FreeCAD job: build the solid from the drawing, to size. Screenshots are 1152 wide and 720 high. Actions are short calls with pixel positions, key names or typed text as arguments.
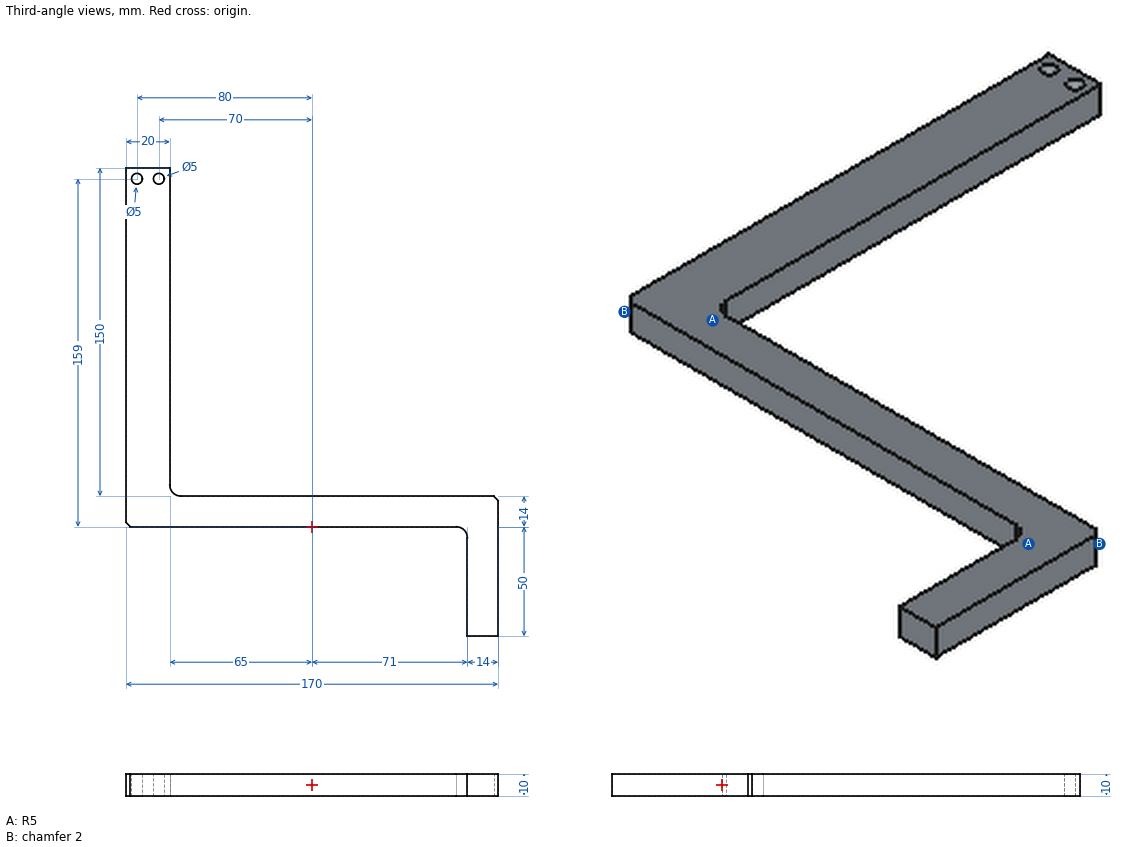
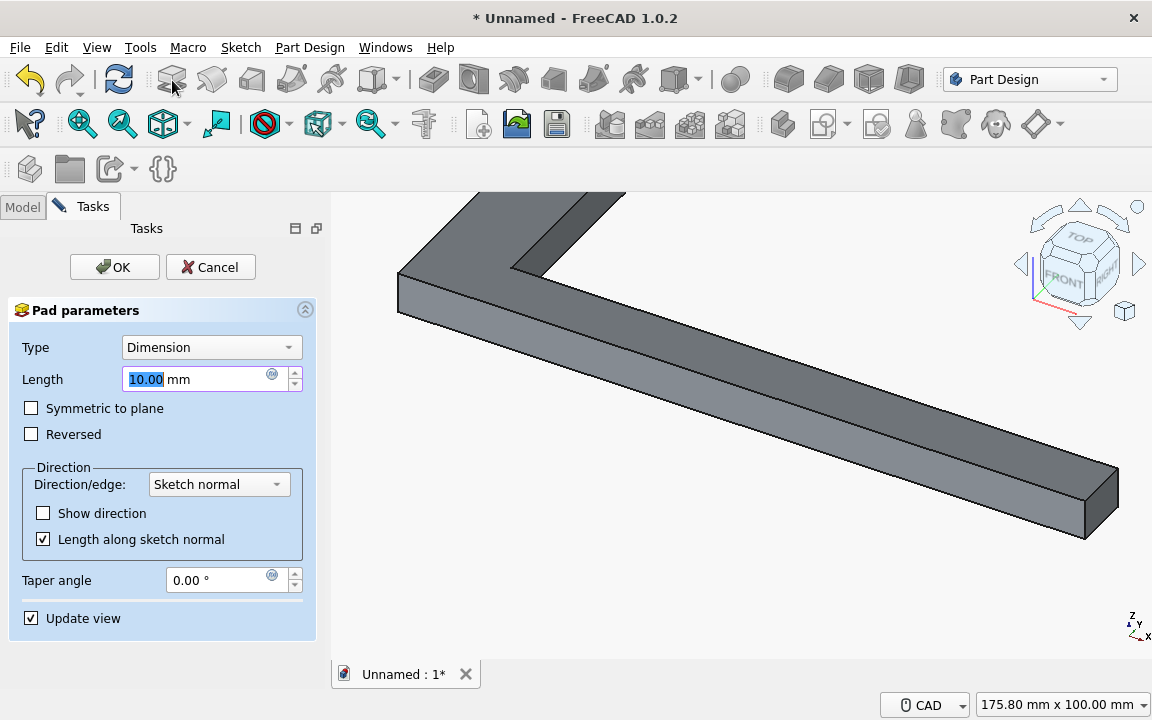
text(10)
key(Tab)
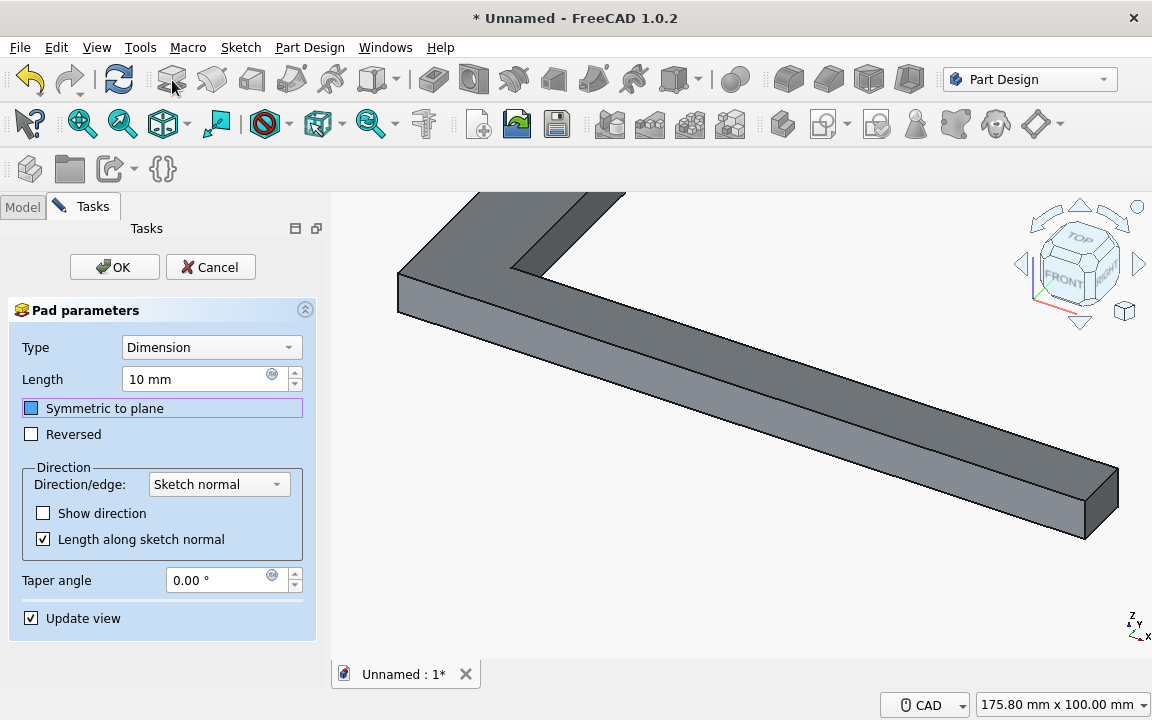
click(30, 408)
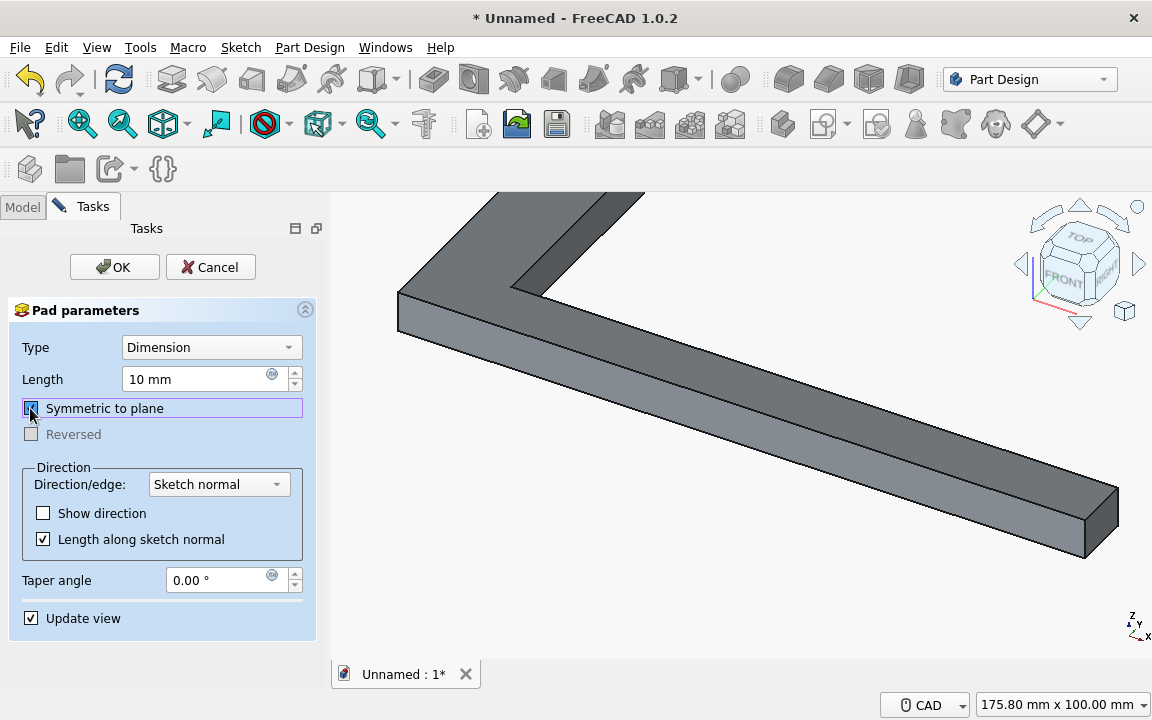
click(115, 267)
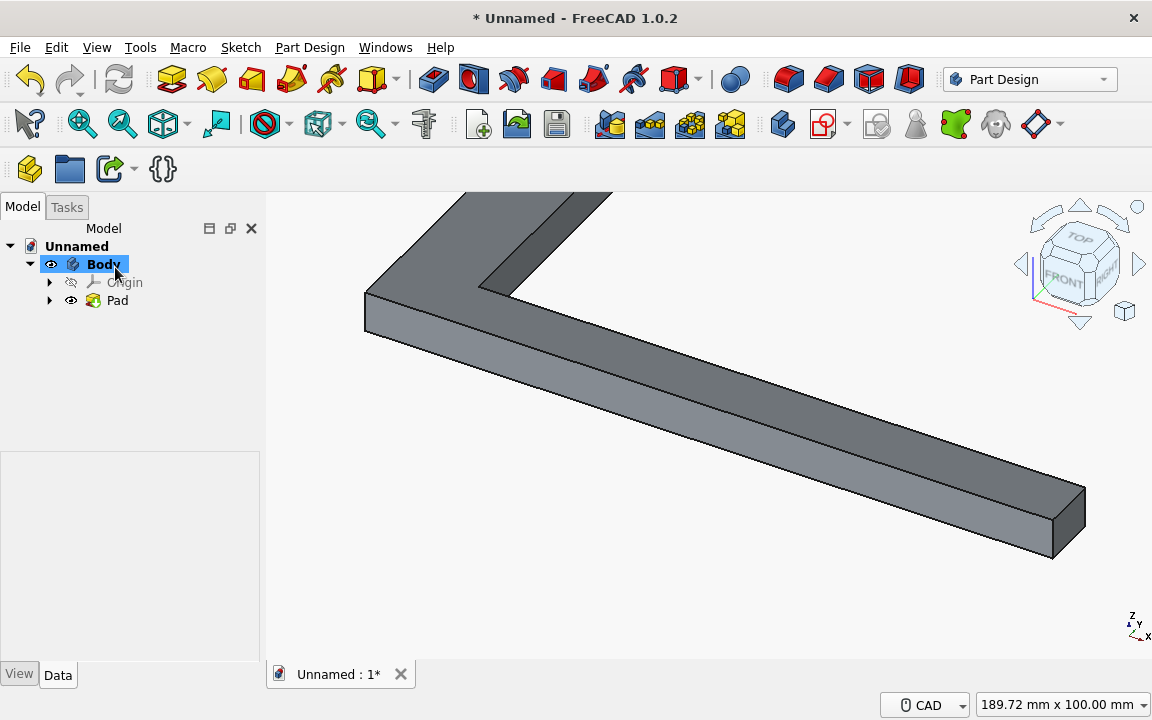
click(84, 124)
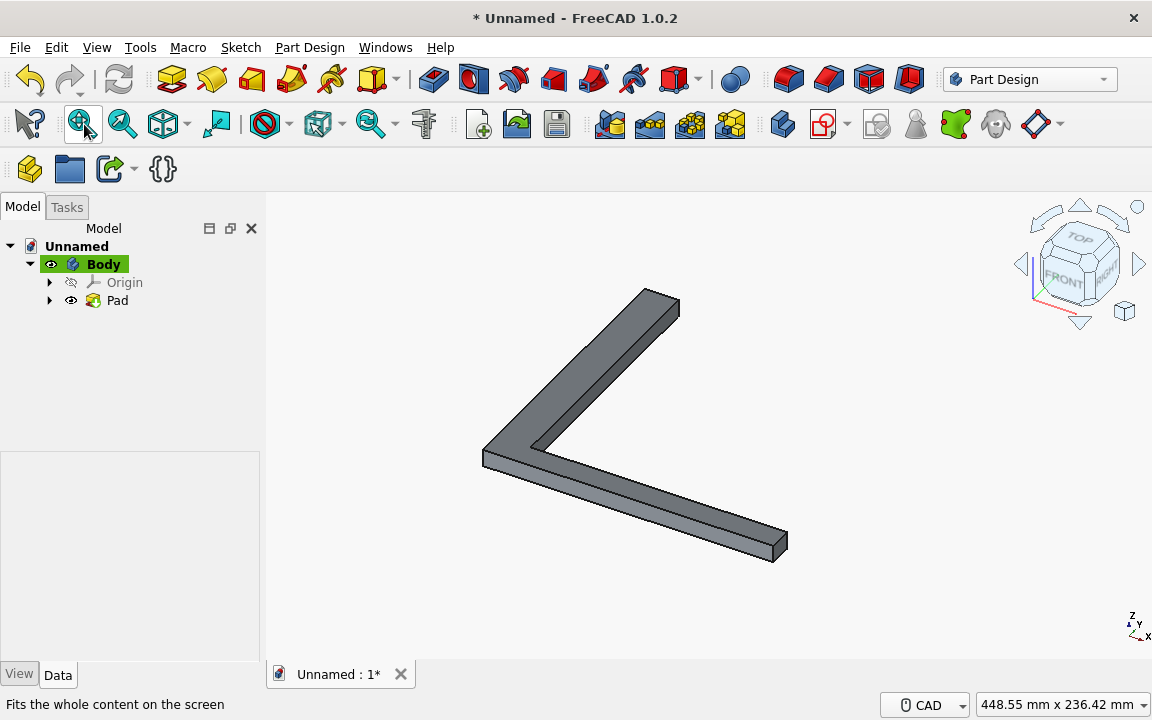
click(515, 444)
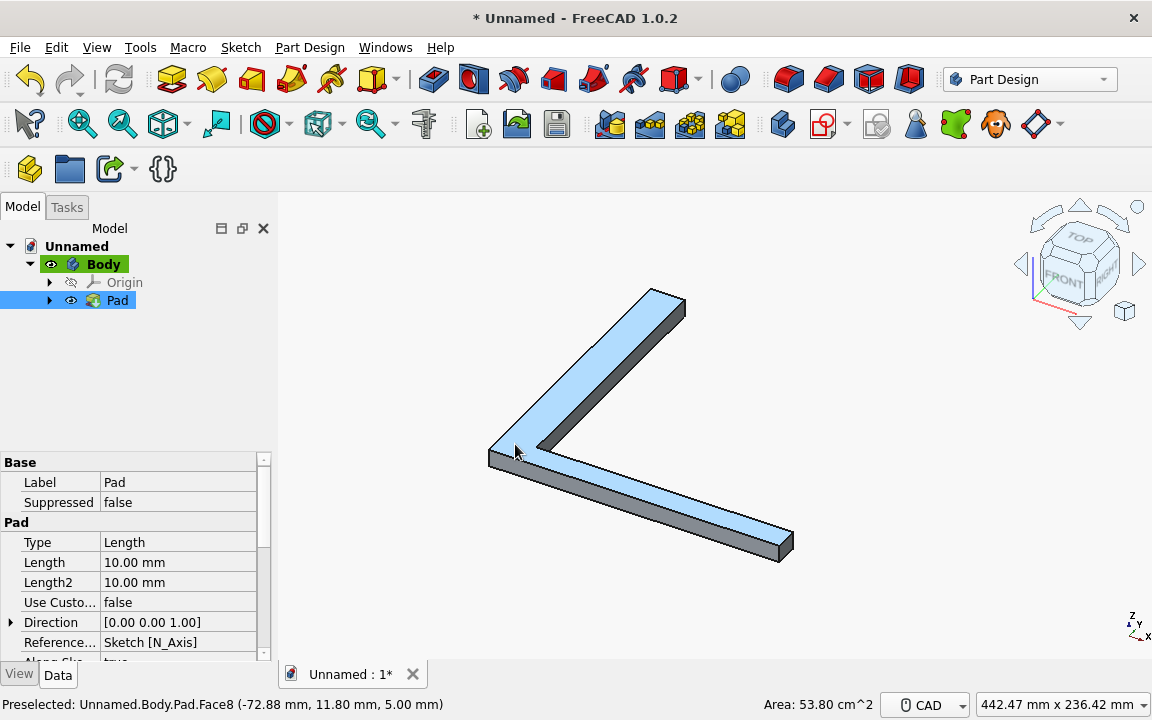
click(824, 124)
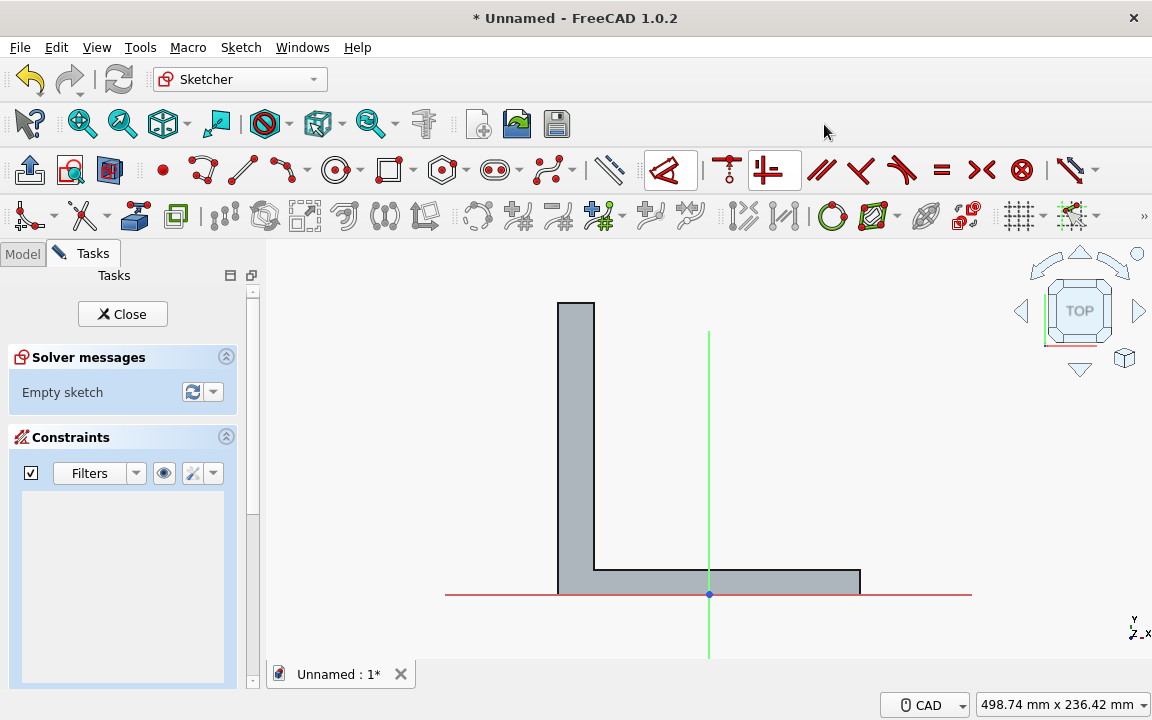
scroll(563, 305, up, 15)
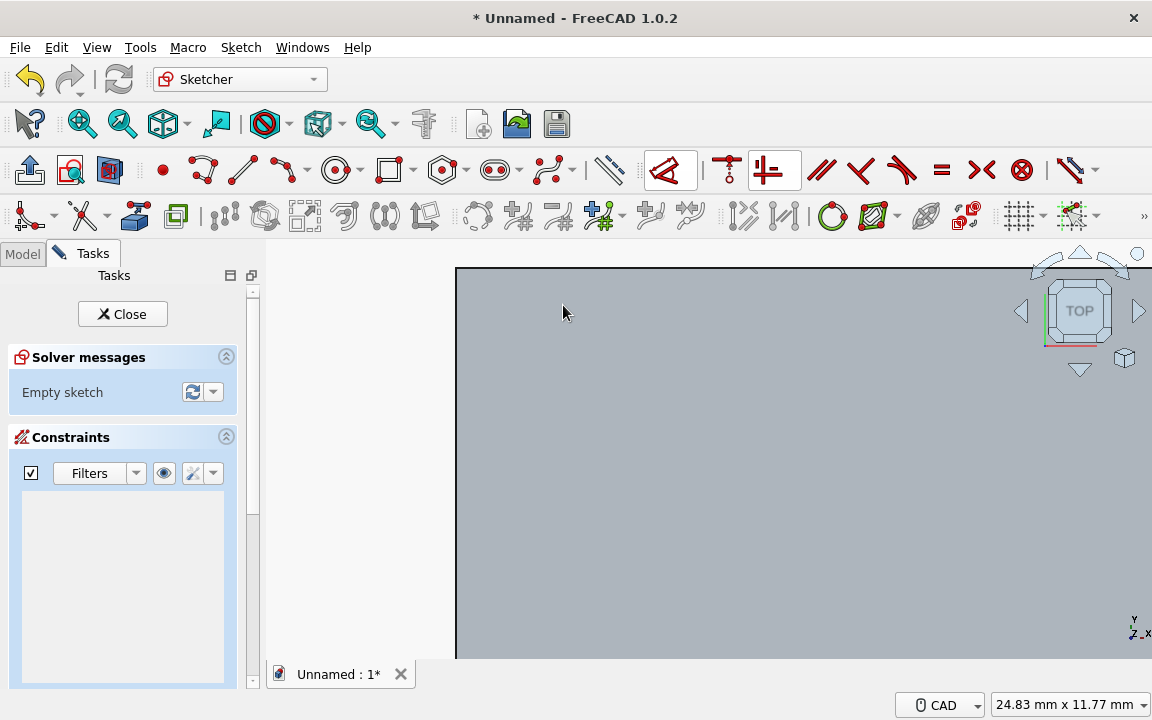
scroll(623, 442, up, 2)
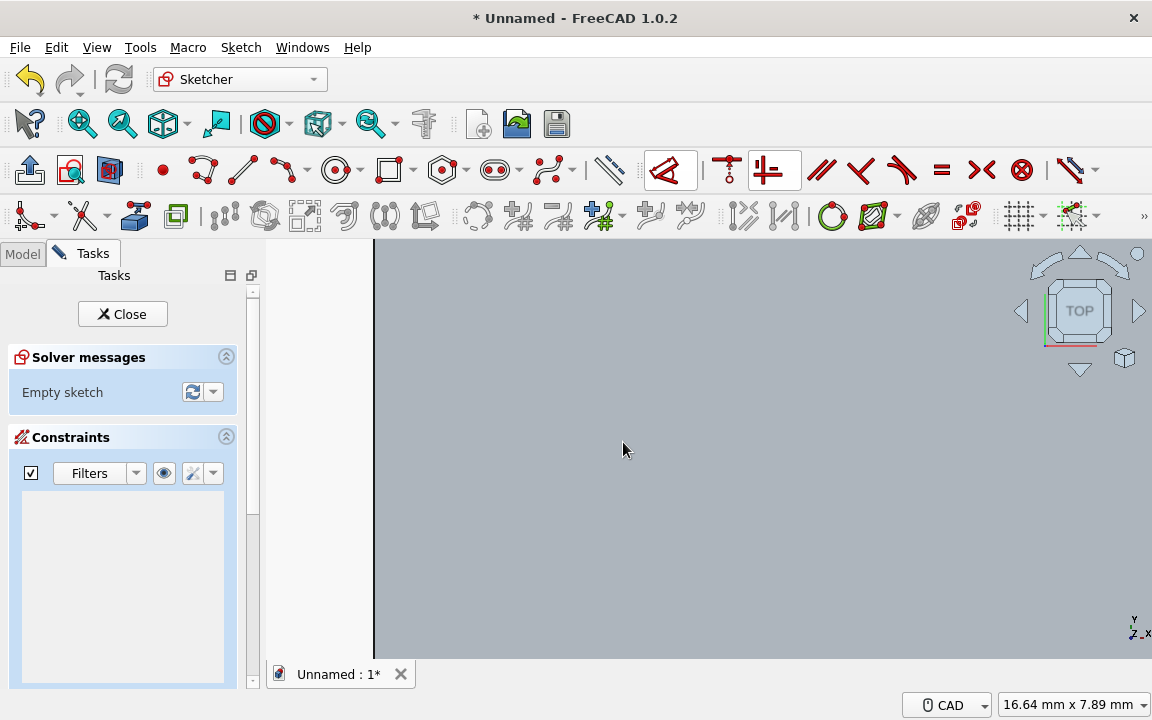
key(g)
key(c)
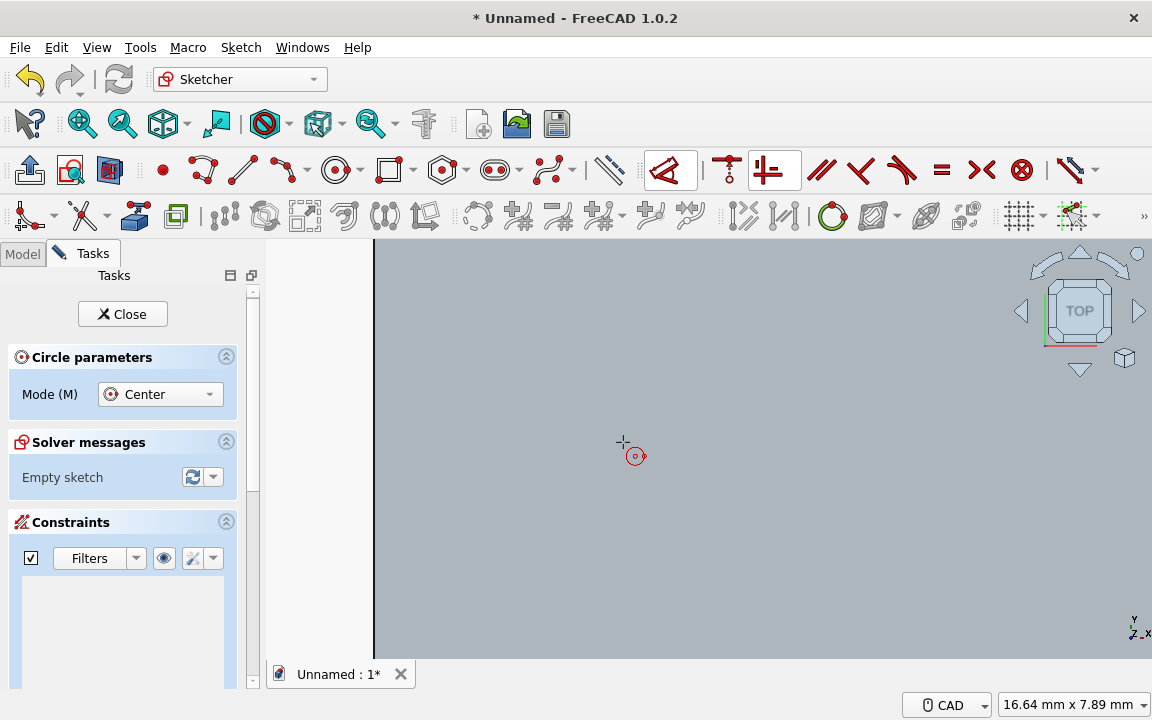
click(640, 449)
move(734, 355)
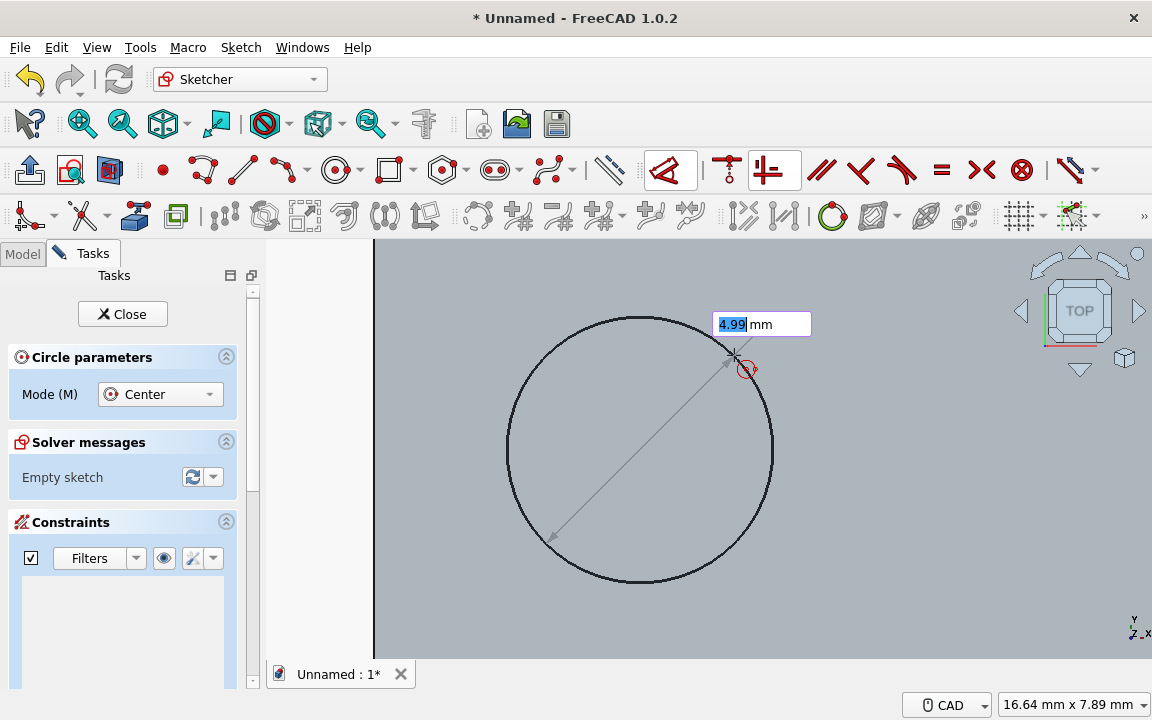
text(5)
key(Return)
key(Escape)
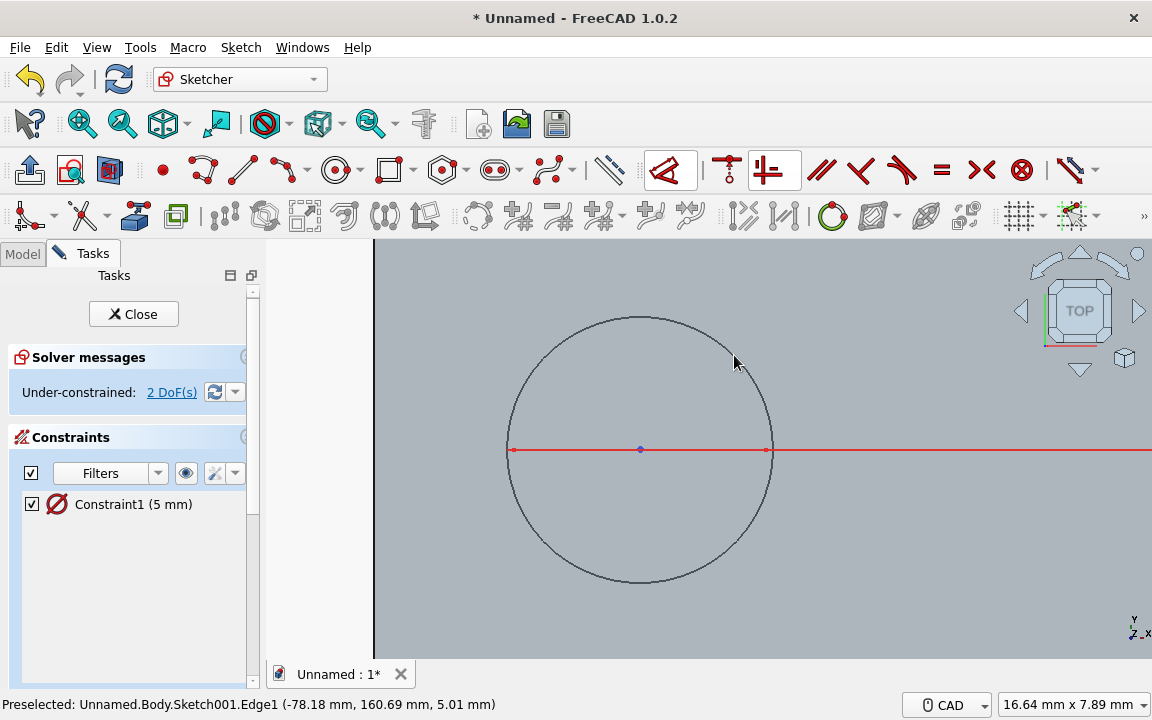
key(d)